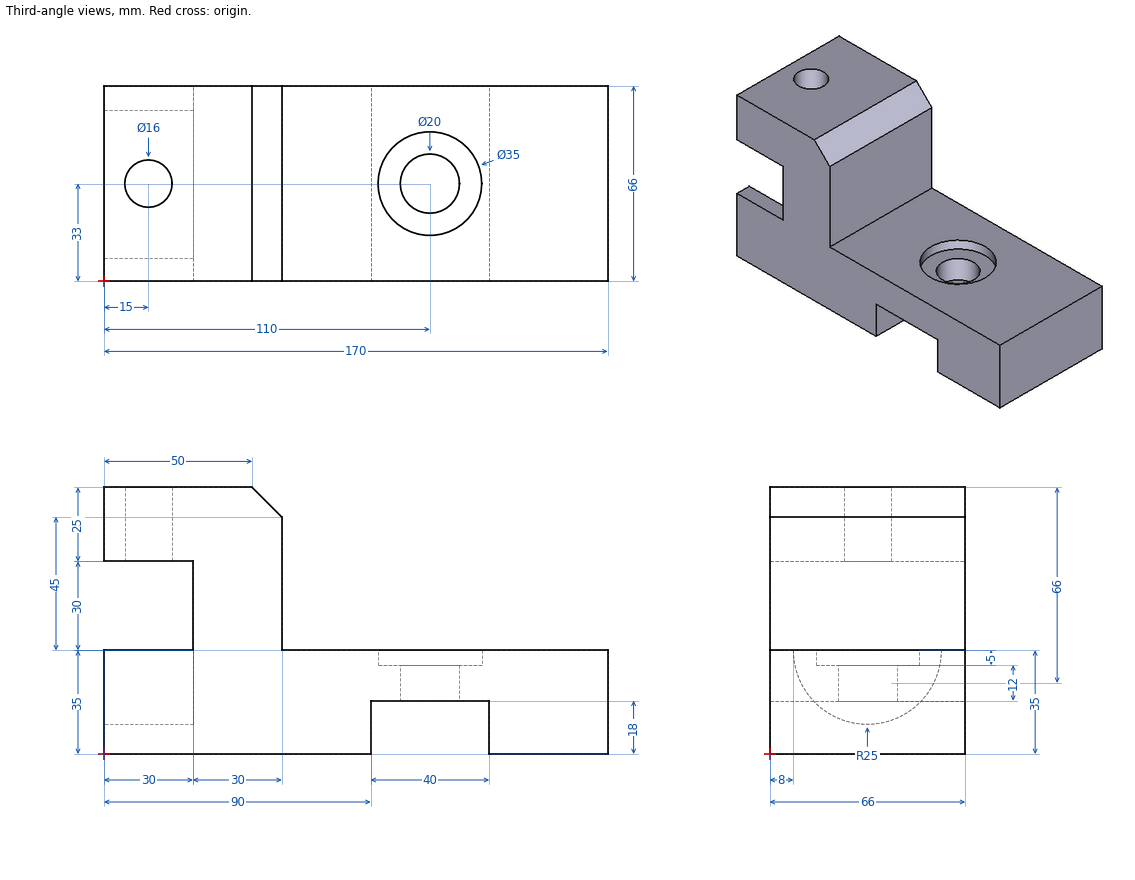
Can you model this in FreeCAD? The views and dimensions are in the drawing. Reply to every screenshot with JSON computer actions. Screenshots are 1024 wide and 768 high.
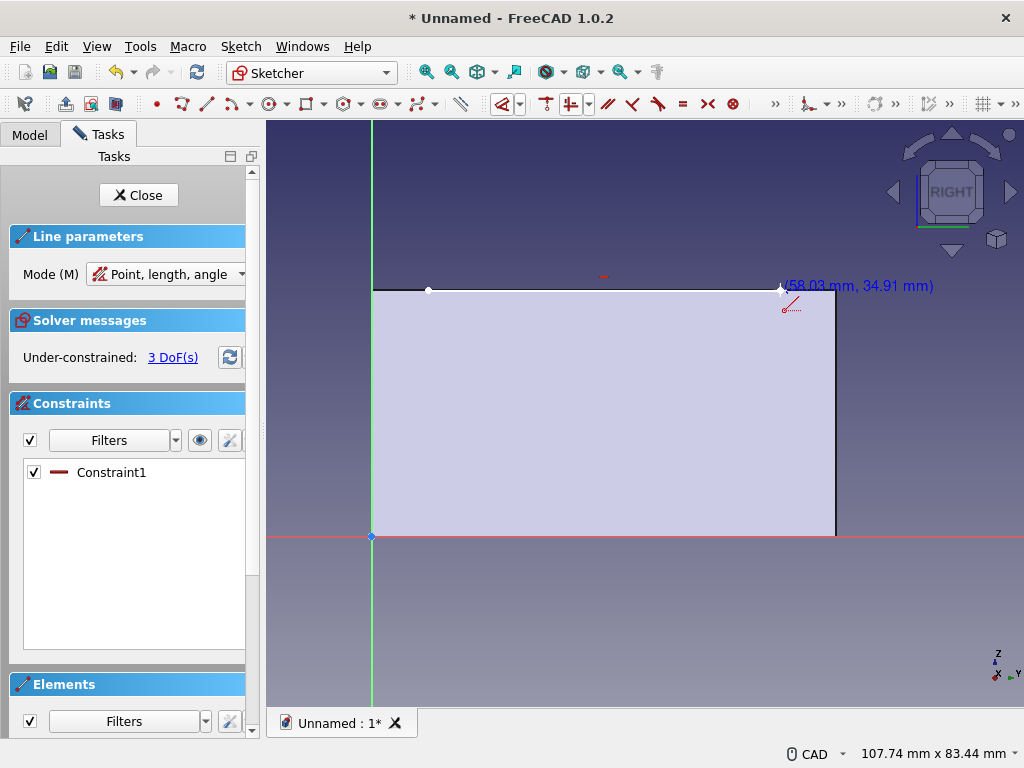
{"action": "key", "text": "g 3 a"}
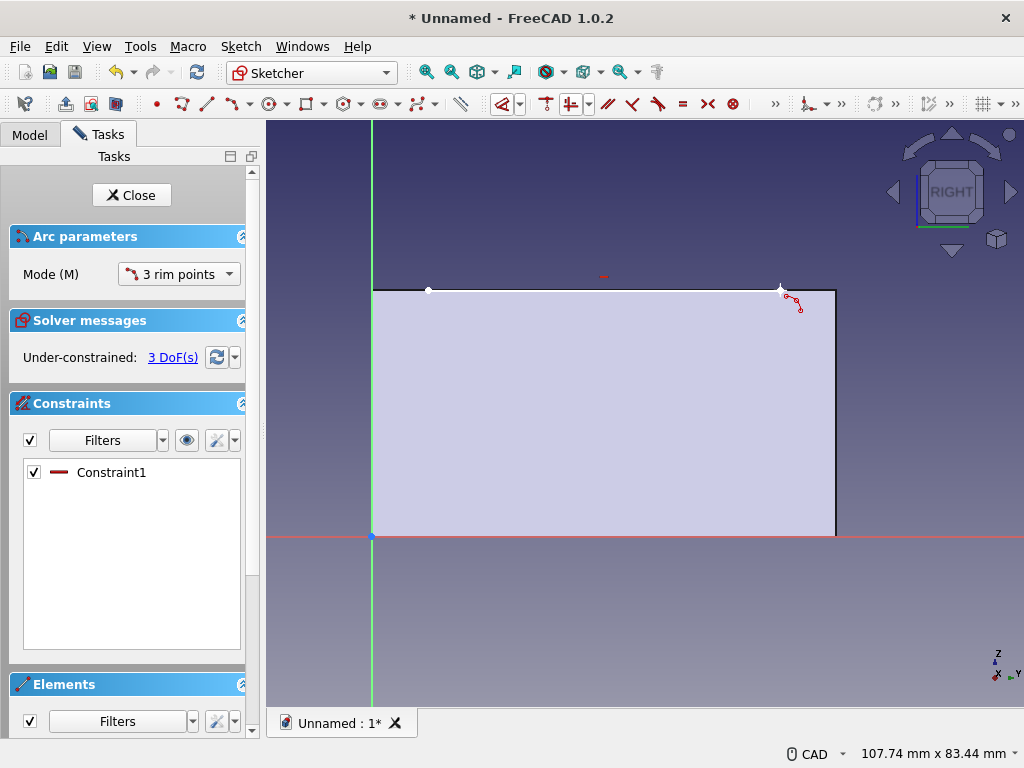
{"action": "left_click", "coordinate": [780, 291]}
{"action": "left_click", "coordinate": [428, 291]}
{"action": "left_click", "coordinate": [604, 466]}
{"action": "key", "text": "Escape"}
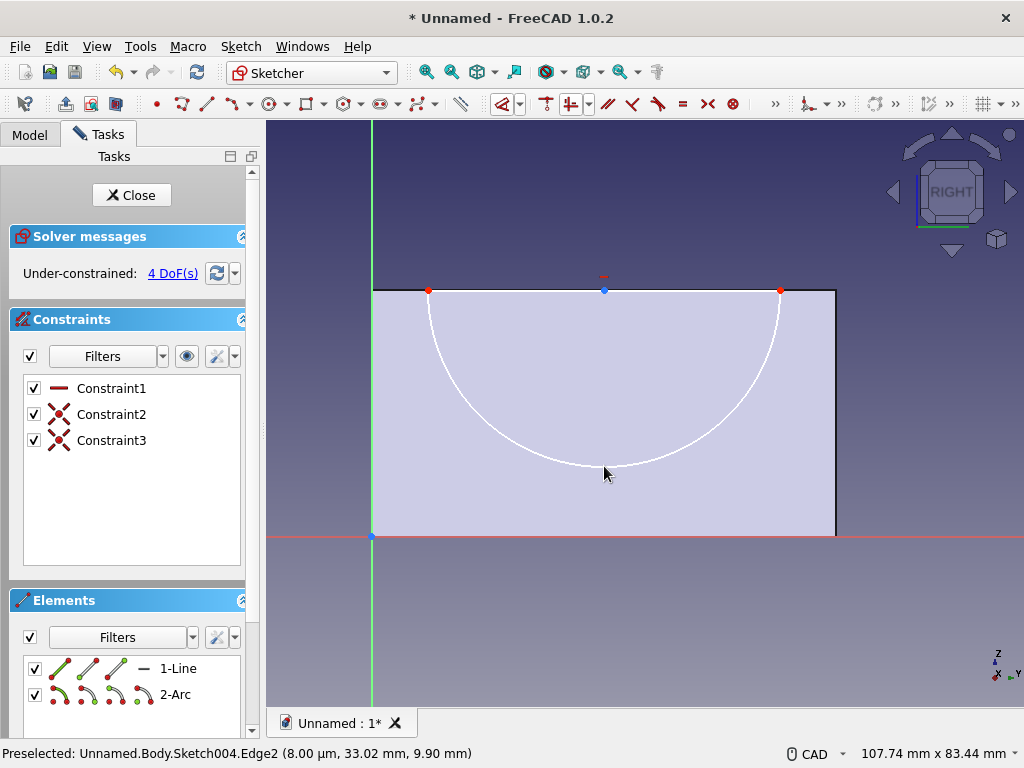
{"action": "left_click", "coordinate": [501, 433]}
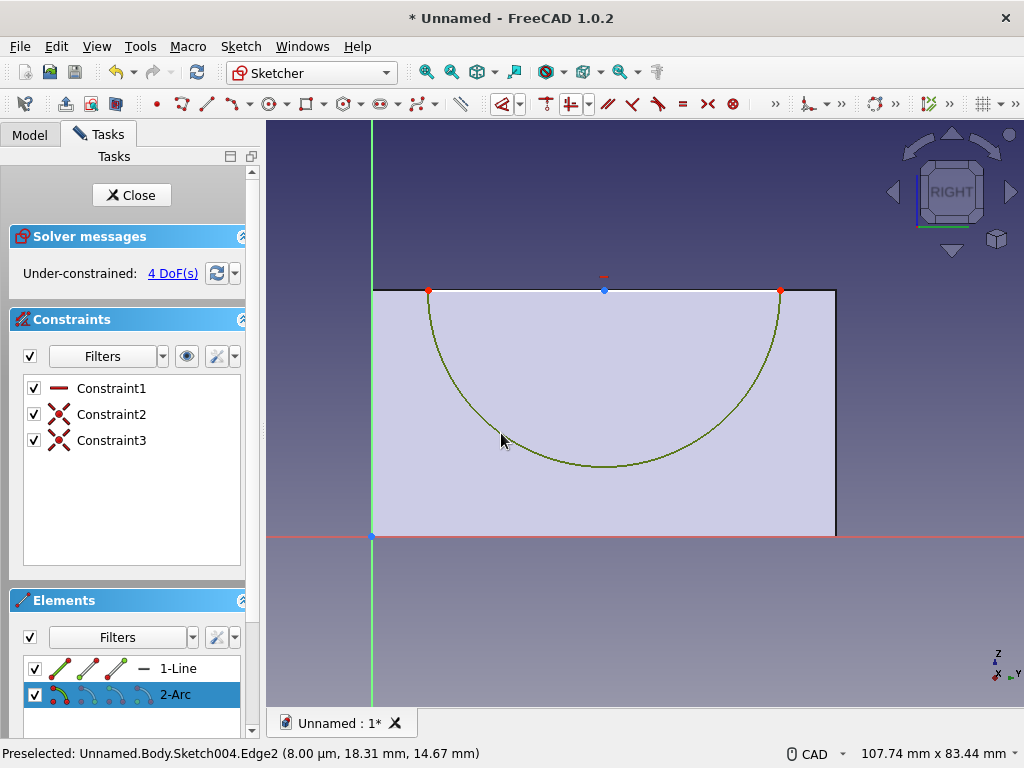
{"action": "key", "text": "k r"}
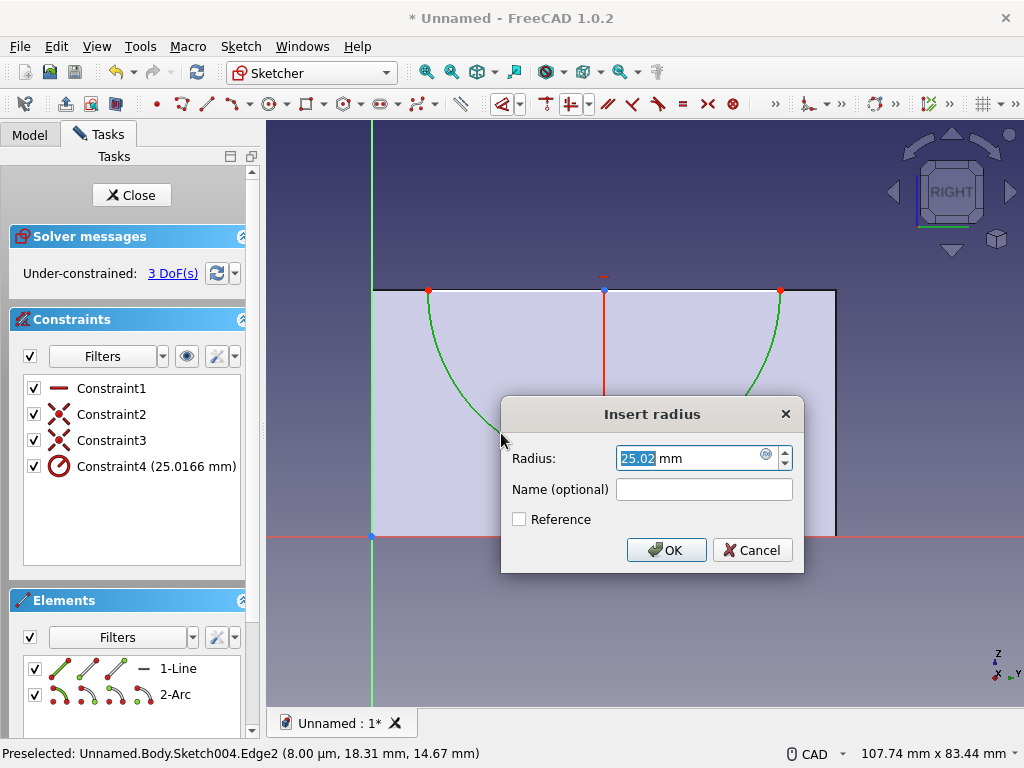
{"action": "type", "text": "25"}
{"action": "key", "text": "Return"}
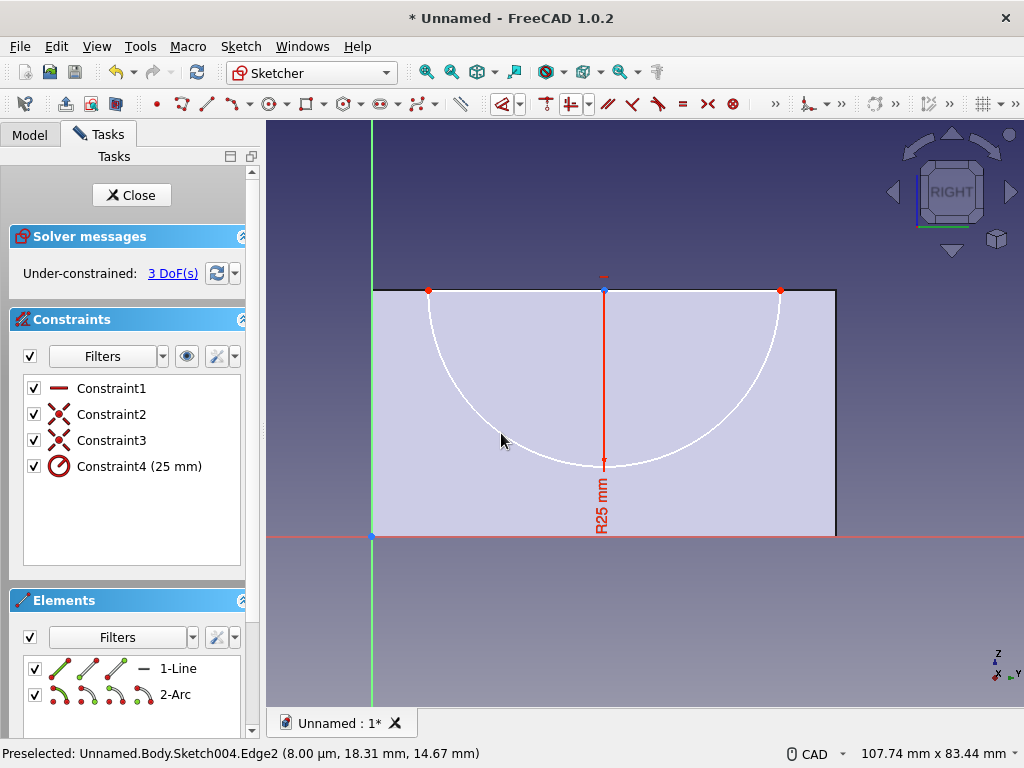
{"action": "left_click", "coordinate": [428, 291]}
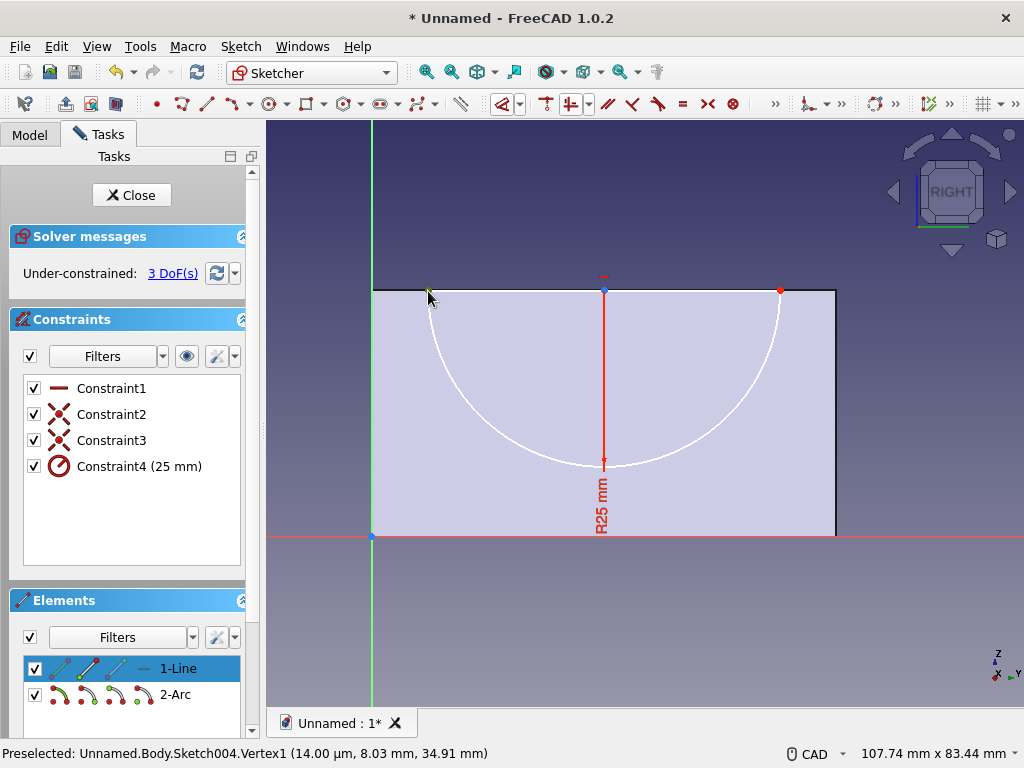
{"action": "key", "text": "l"}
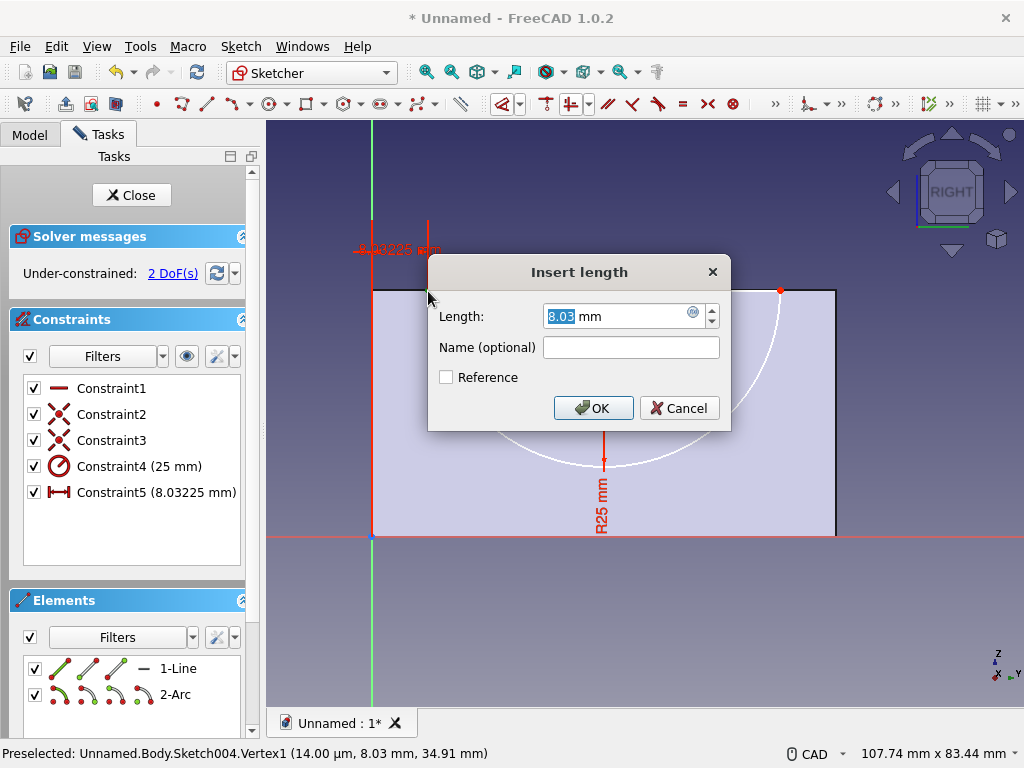
{"action": "type", "text": "8"}
{"action": "key", "text": "Return"}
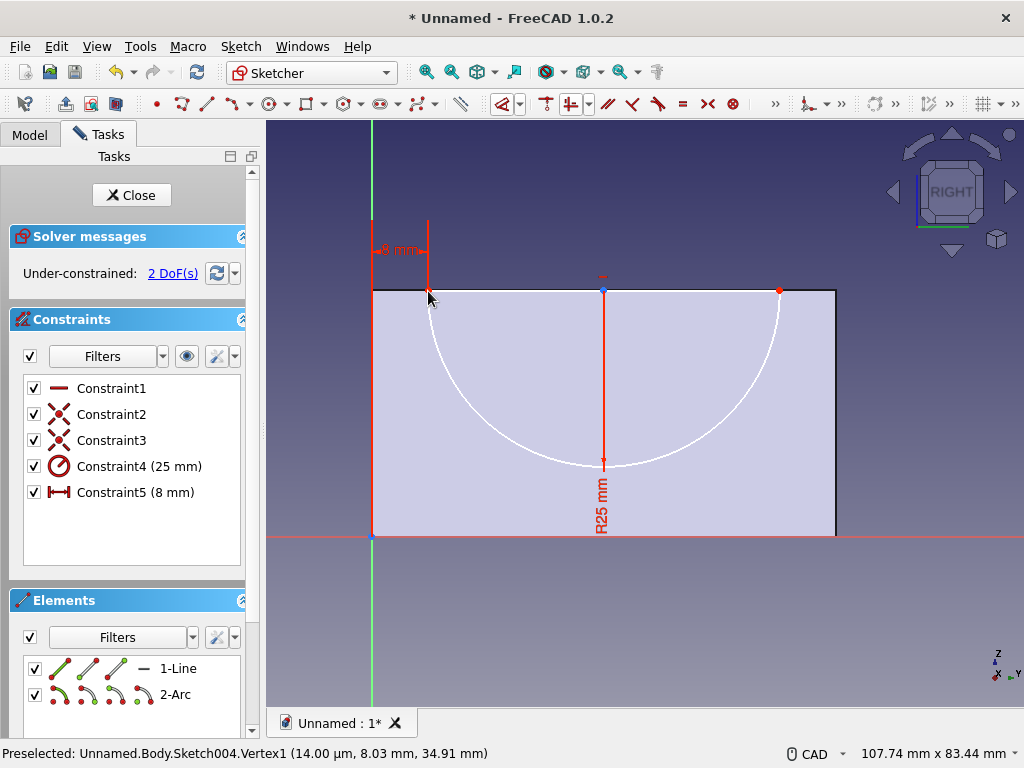
{"action": "left_click", "coordinate": [428, 291]}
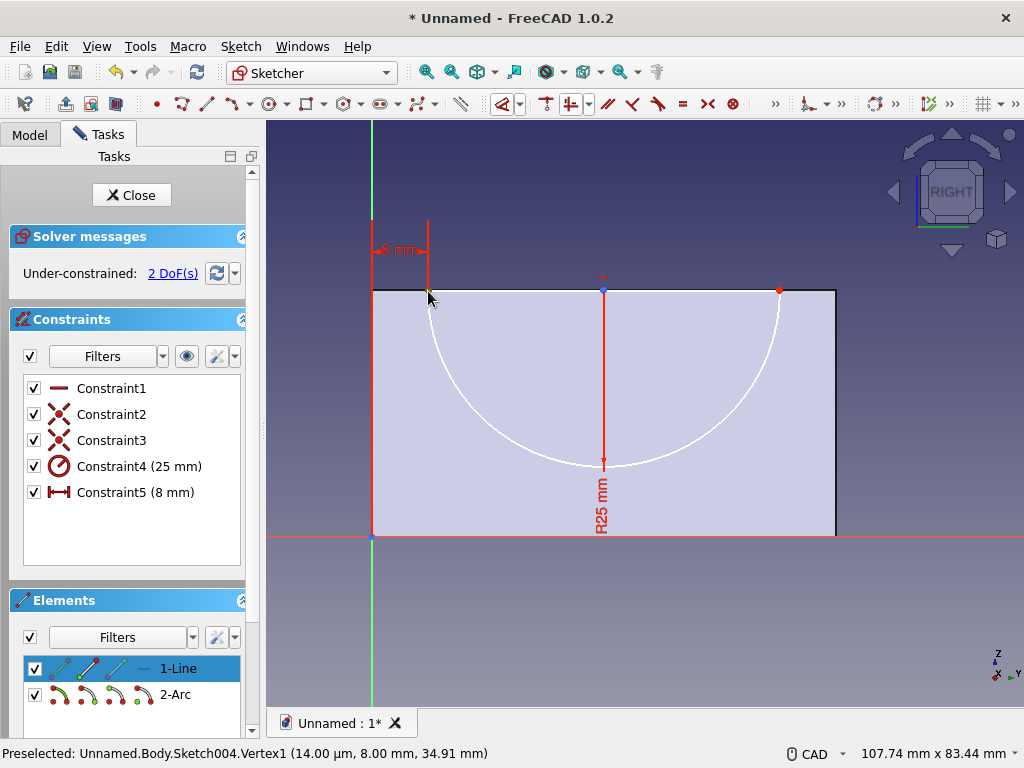
{"action": "key", "text": "i"}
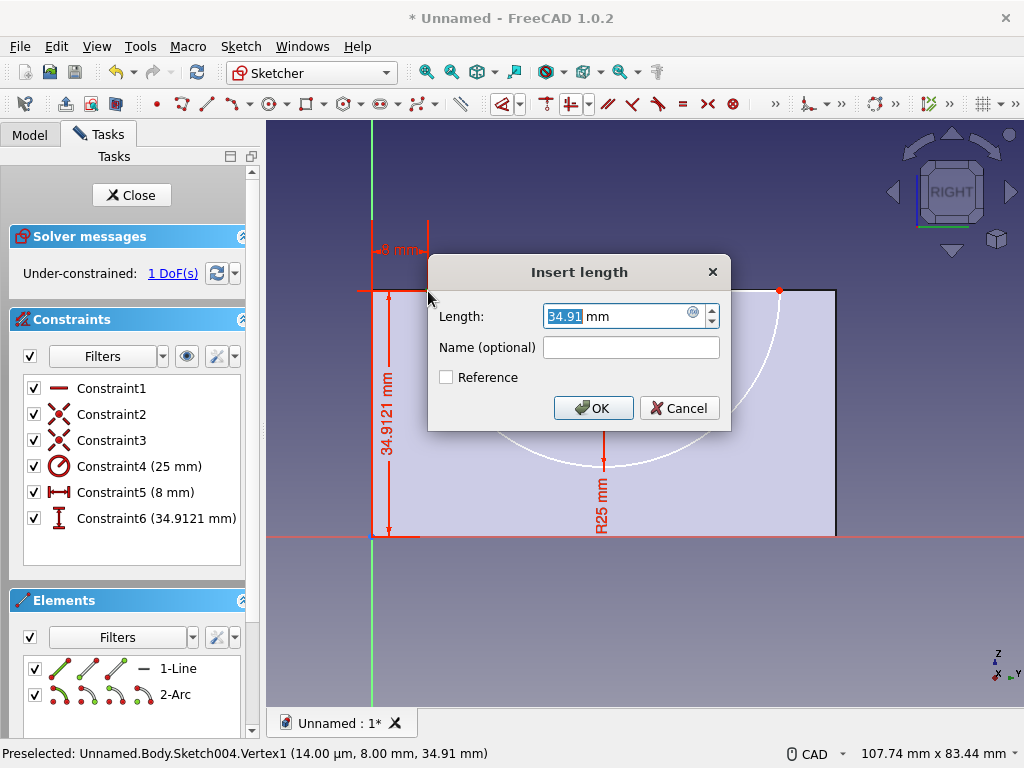
{"action": "type", "text": "35"}
{"action": "key", "text": "Return"}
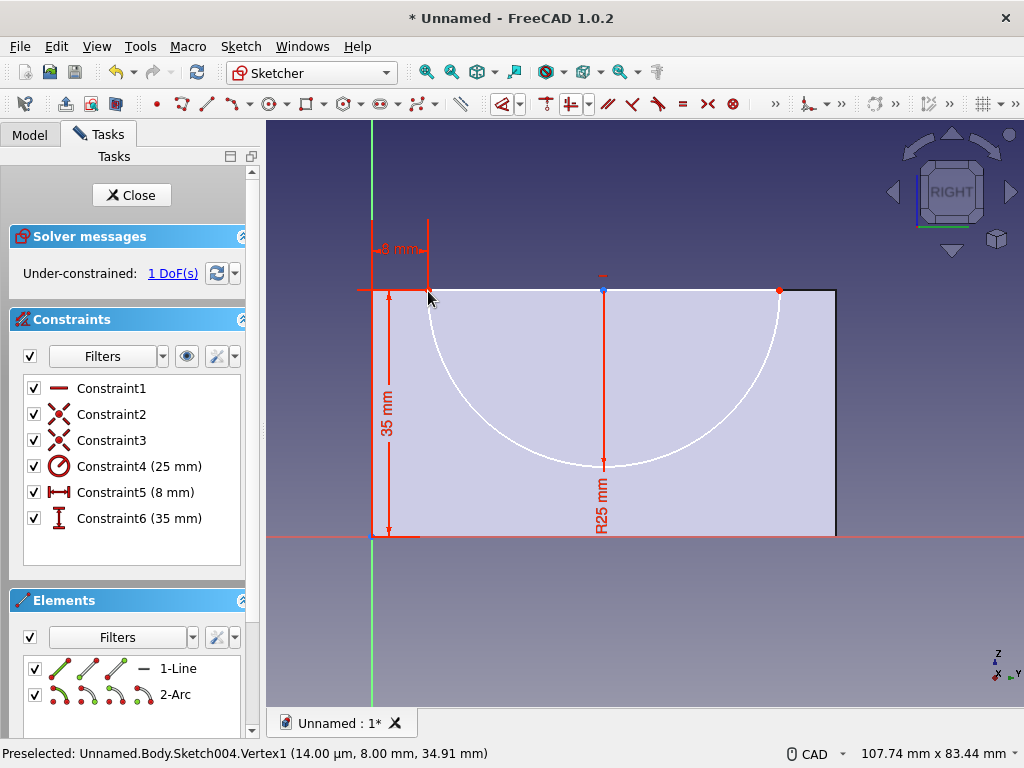
{"action": "left_click", "coordinate": [604, 291]}